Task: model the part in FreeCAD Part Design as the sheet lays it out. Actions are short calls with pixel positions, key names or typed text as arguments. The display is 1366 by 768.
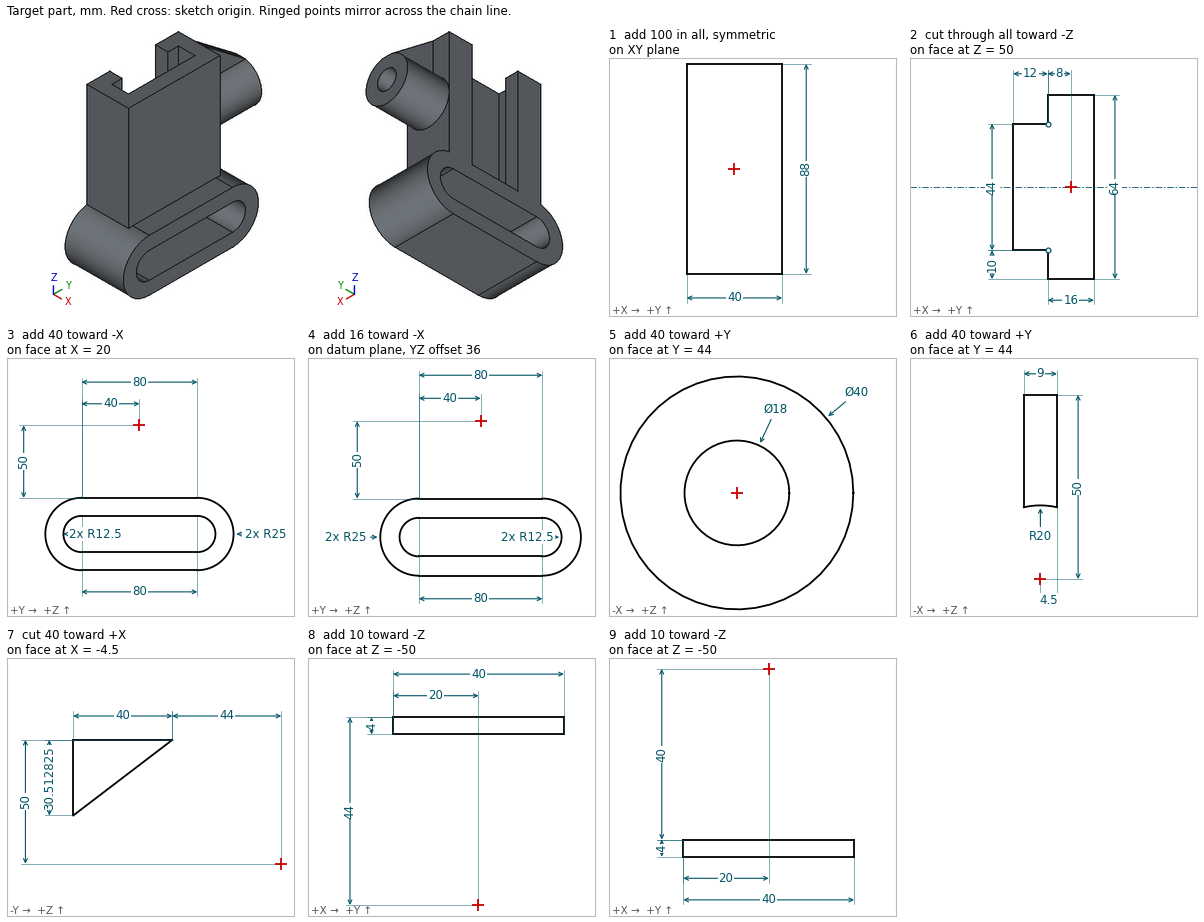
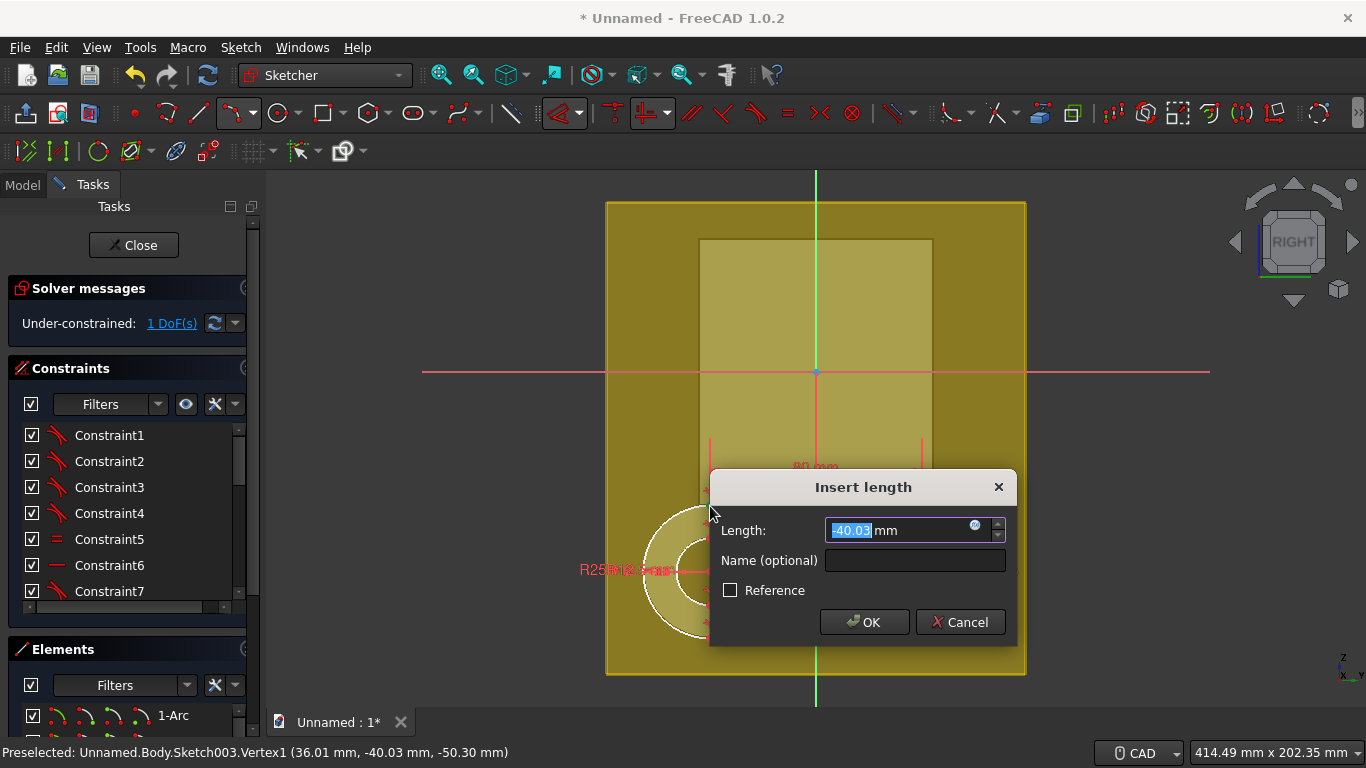
text(-40)
key(Return)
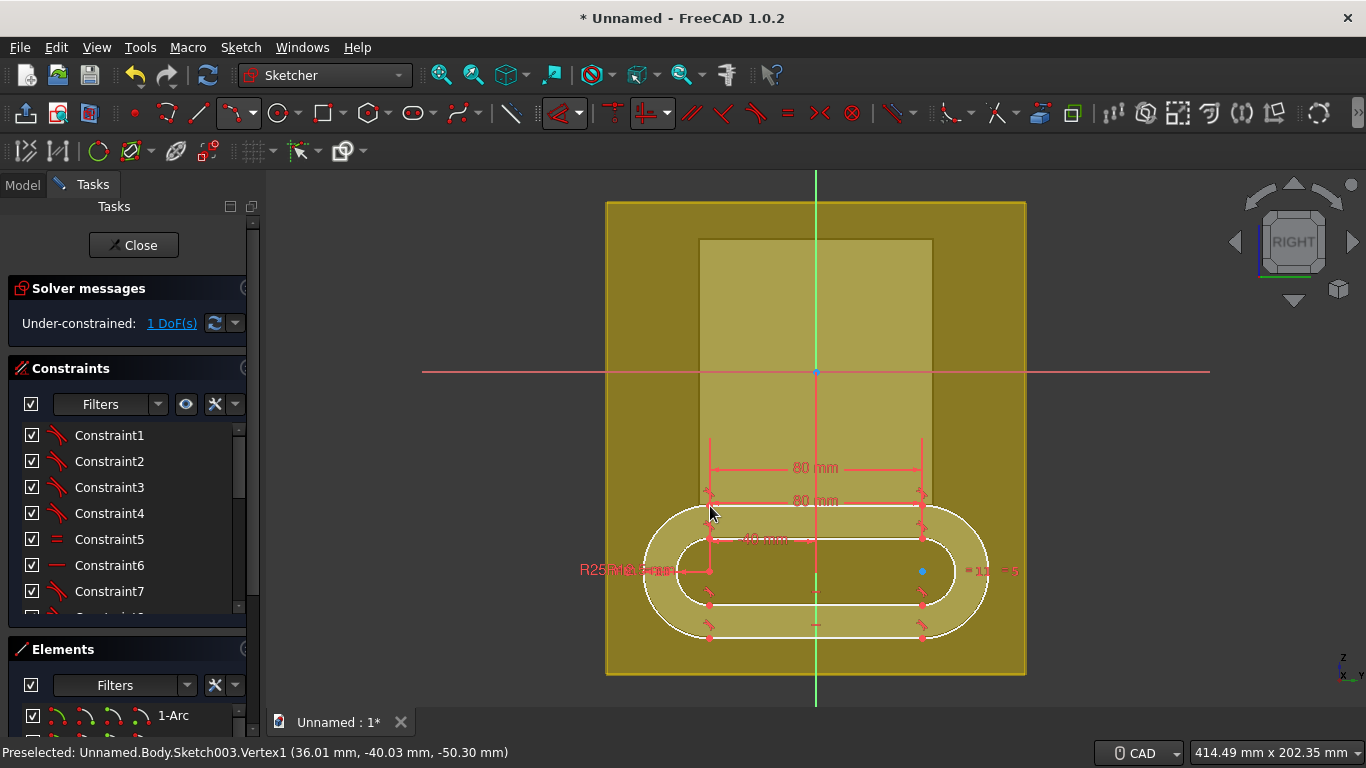
click(710, 506)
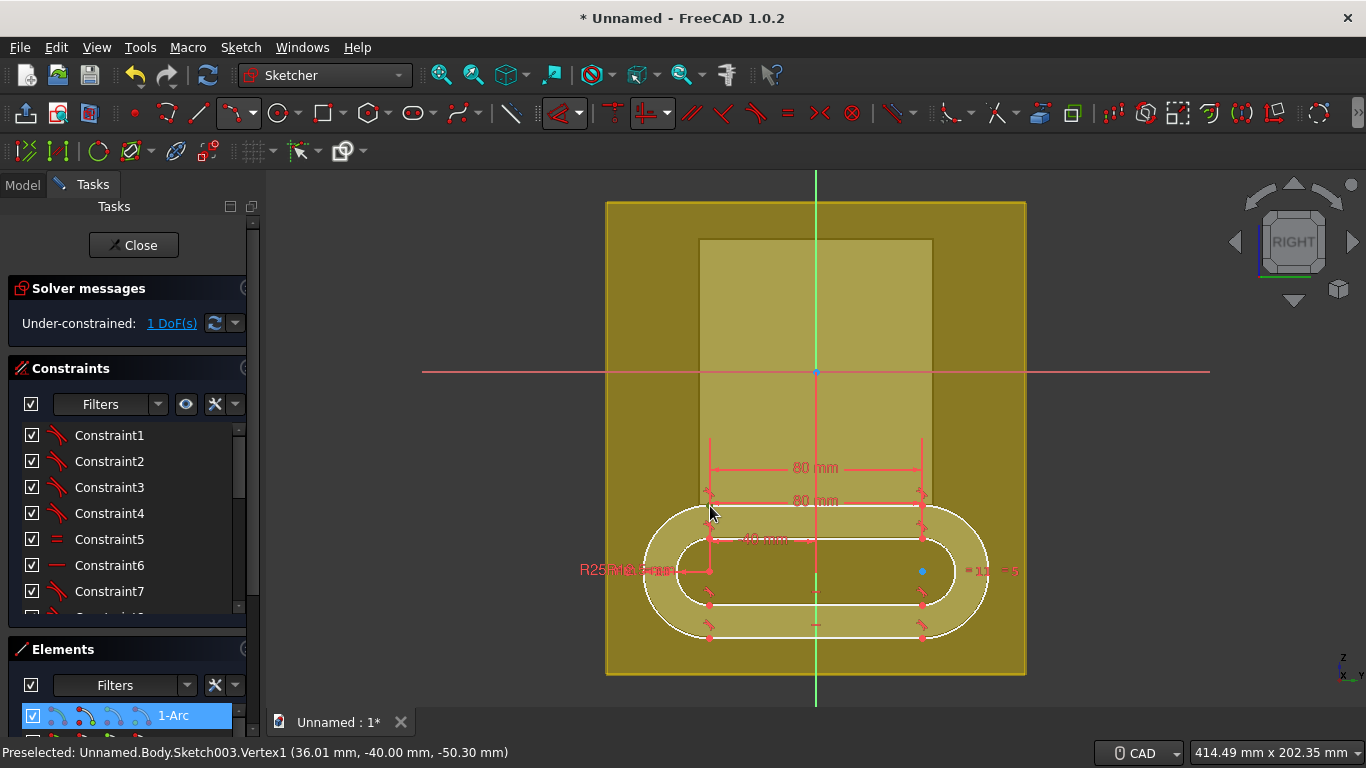
key(i)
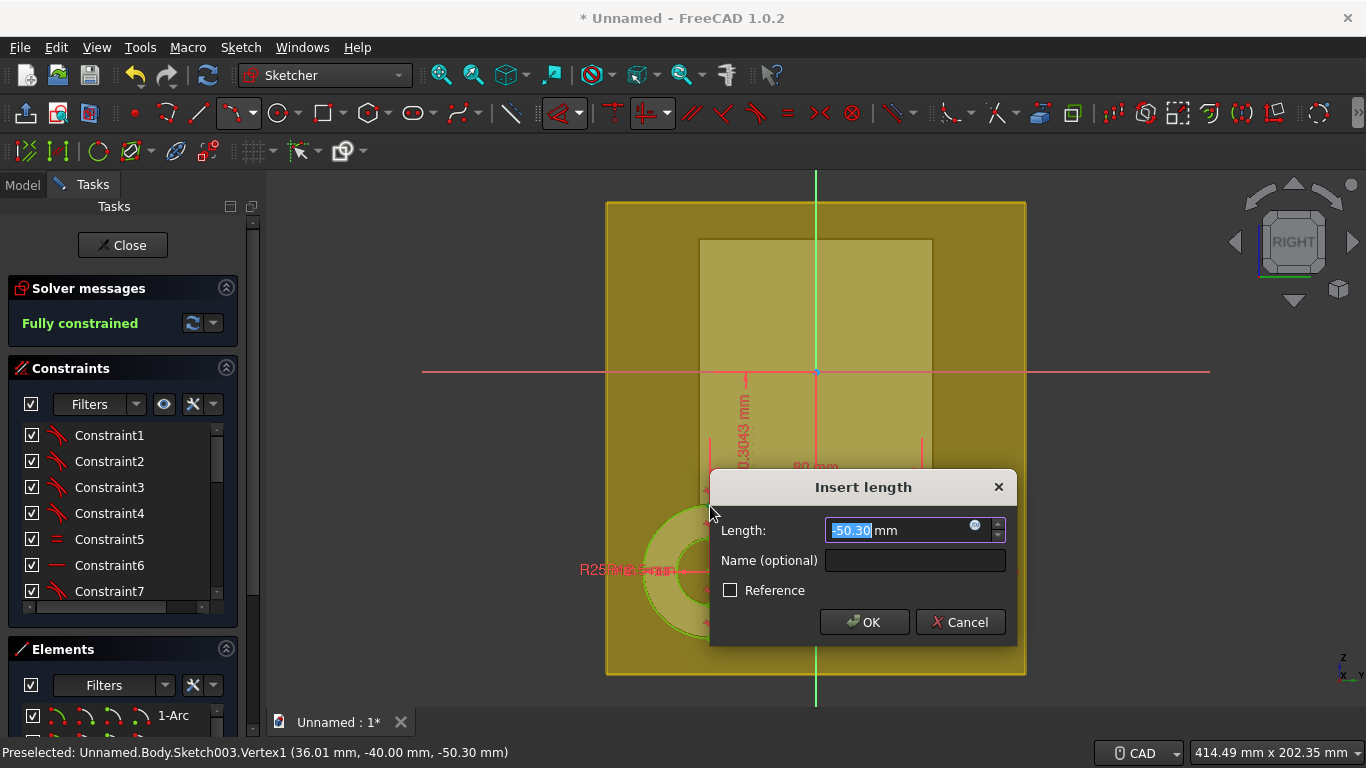
text(-50)
key(Return)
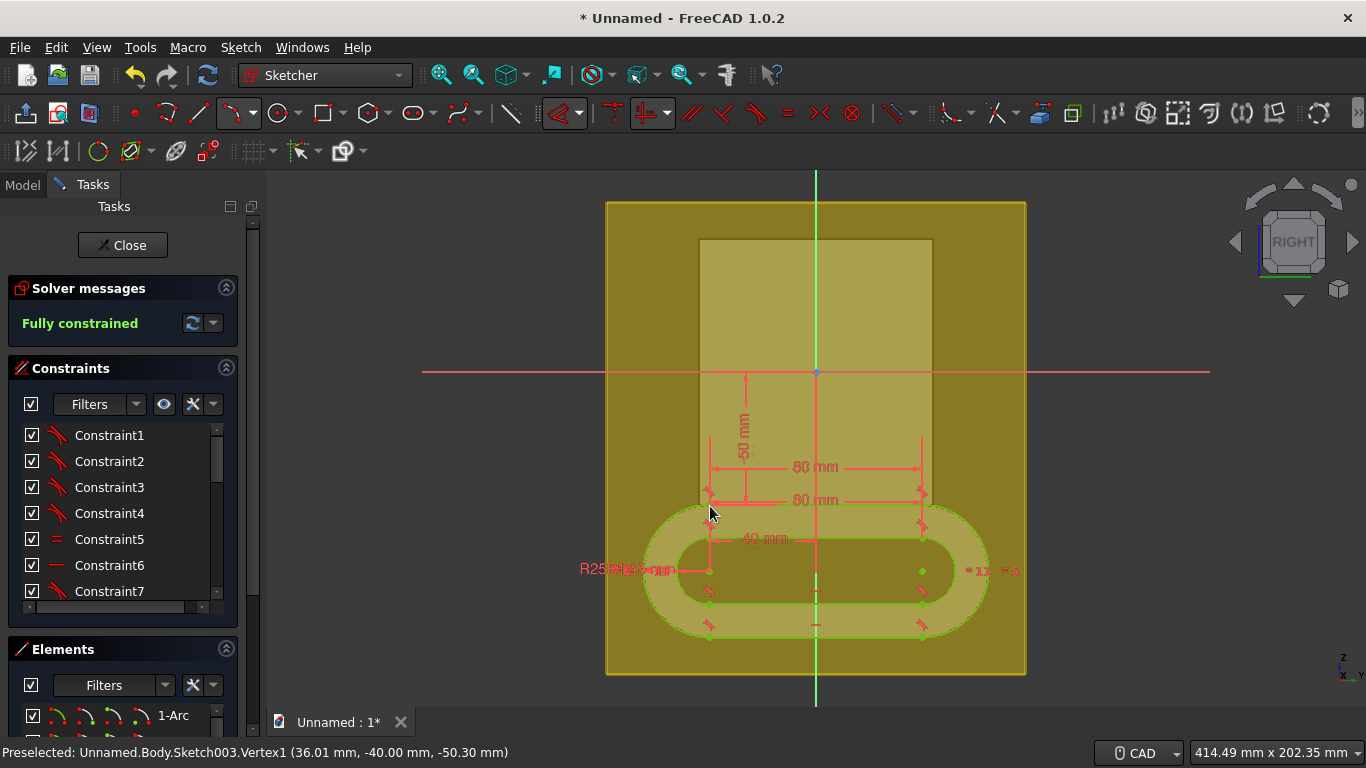
click(123, 245)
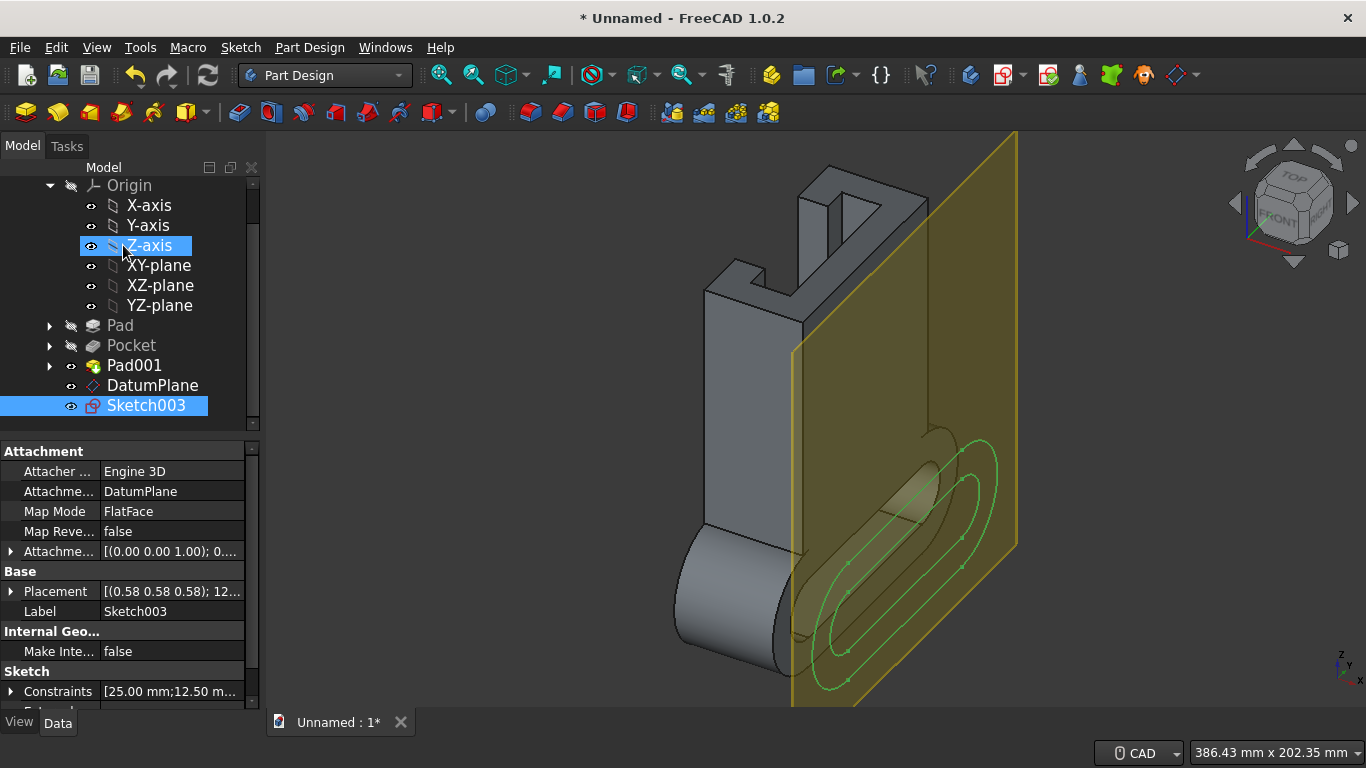
click(26, 112)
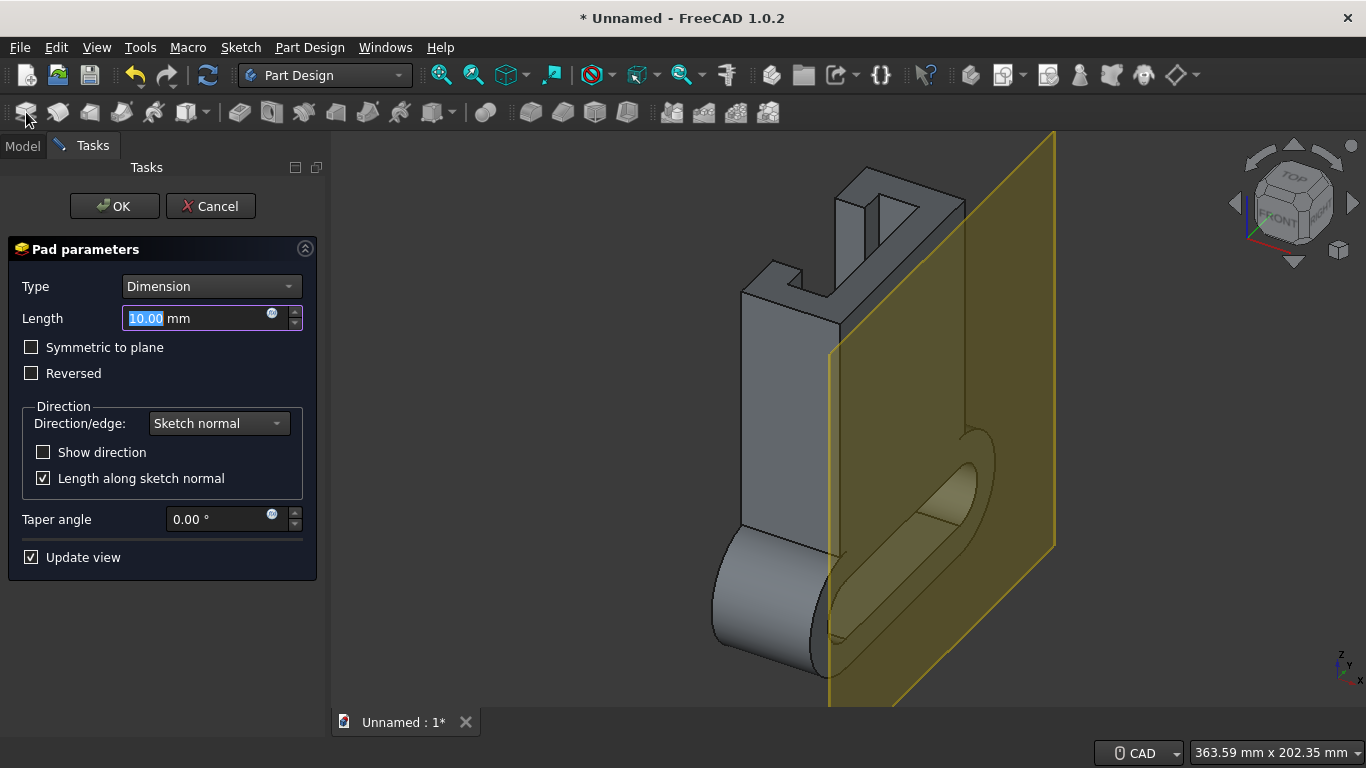
text(16)
key(Tab)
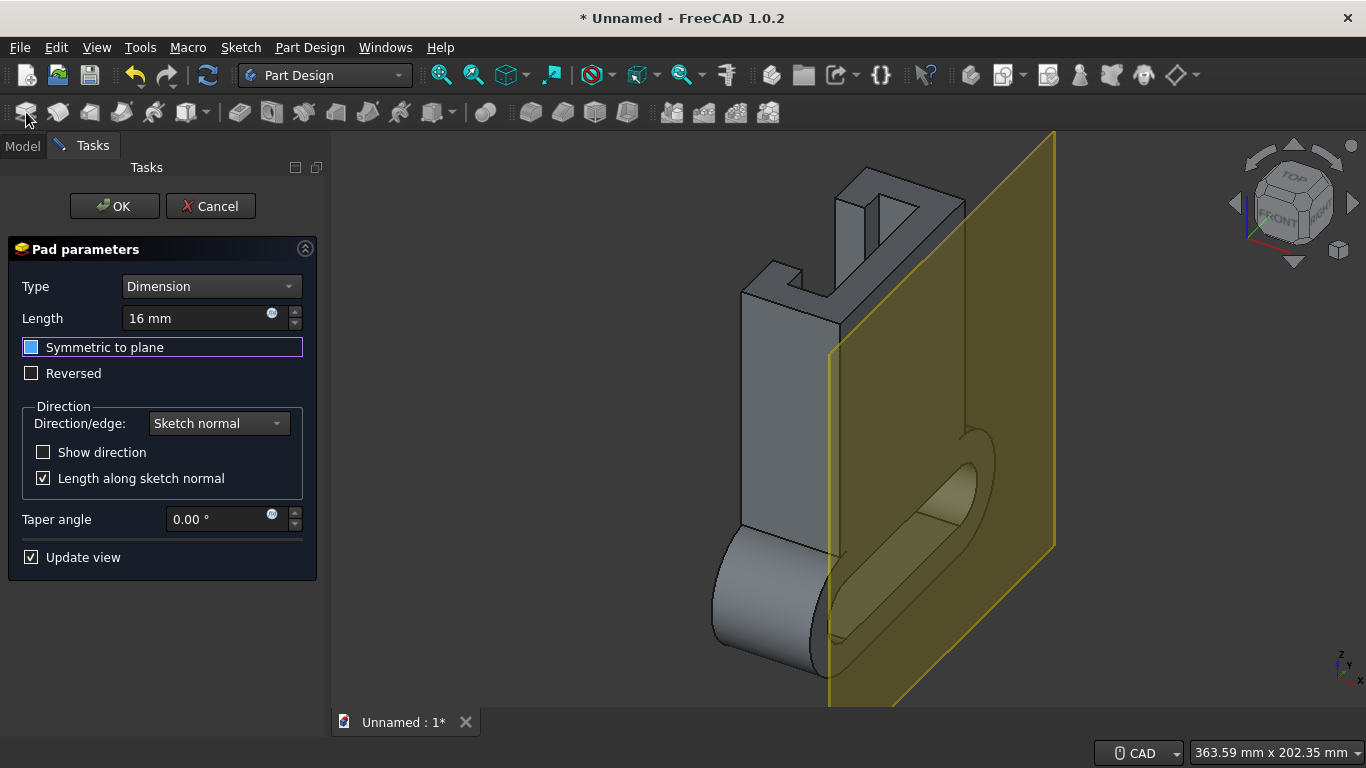
click(30, 373)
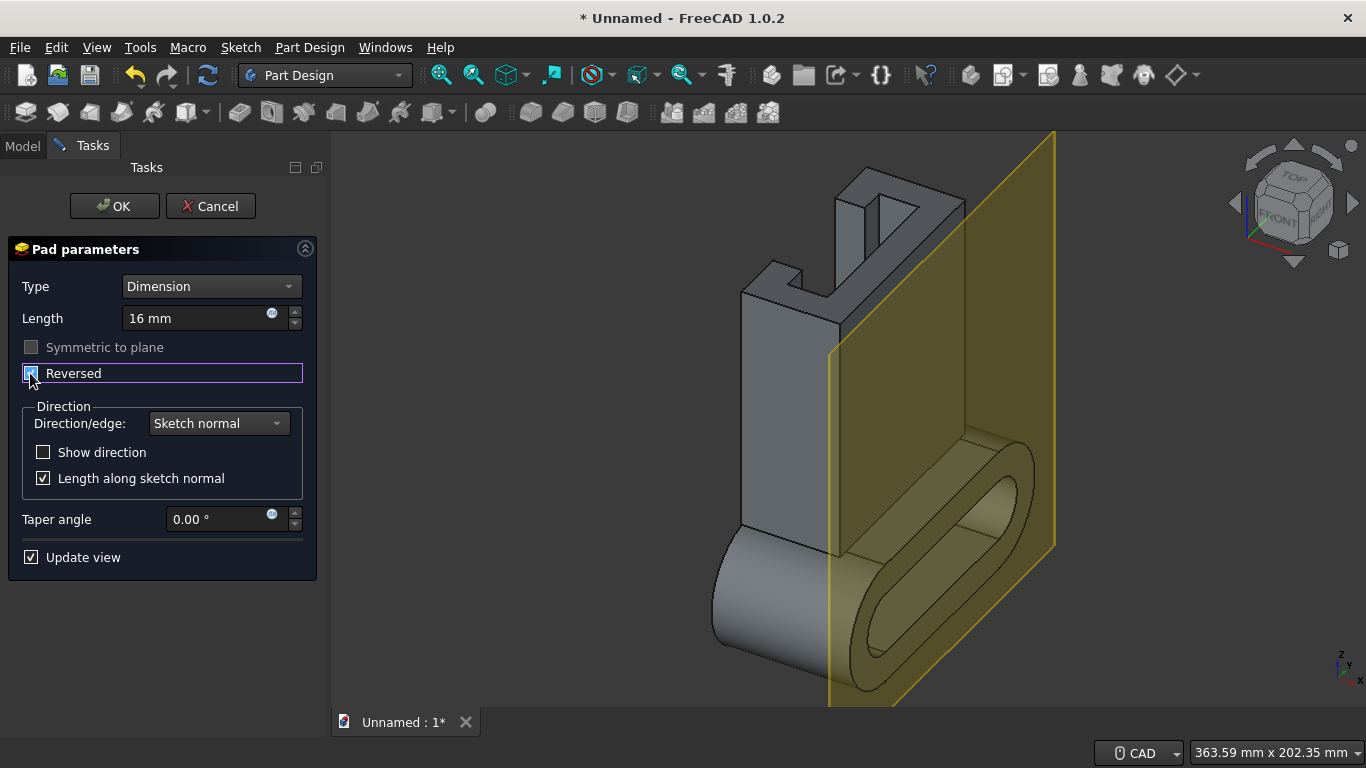
click(115, 206)